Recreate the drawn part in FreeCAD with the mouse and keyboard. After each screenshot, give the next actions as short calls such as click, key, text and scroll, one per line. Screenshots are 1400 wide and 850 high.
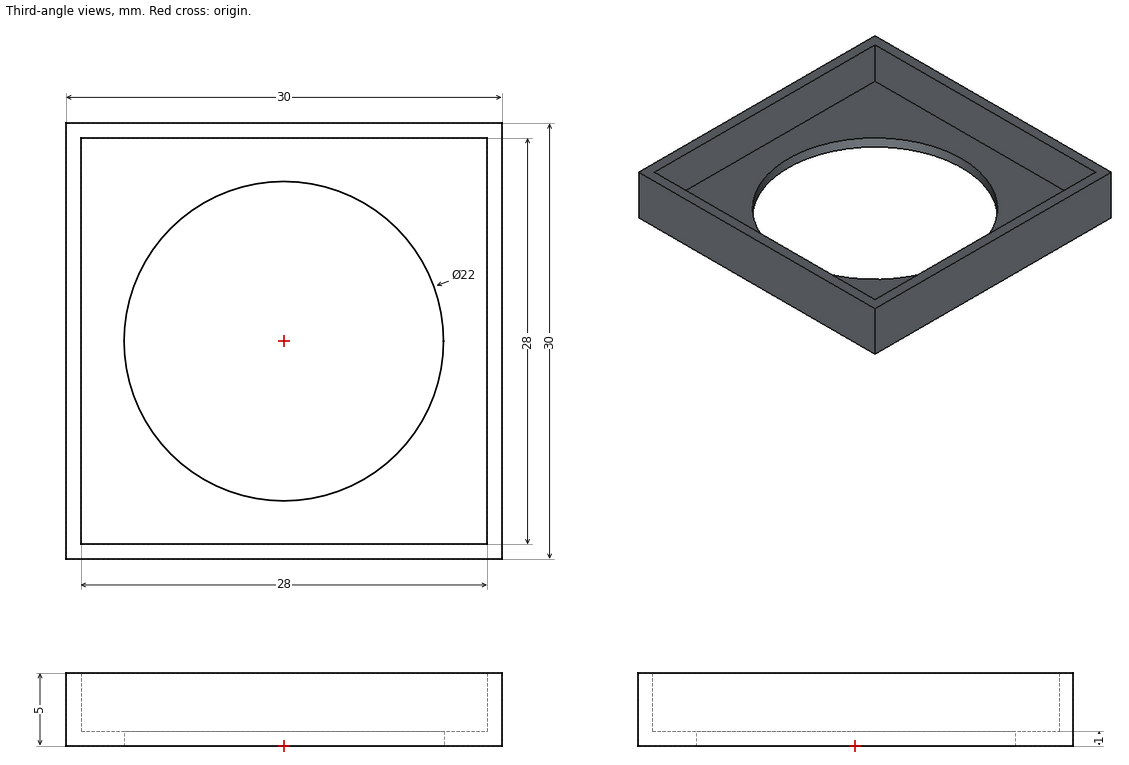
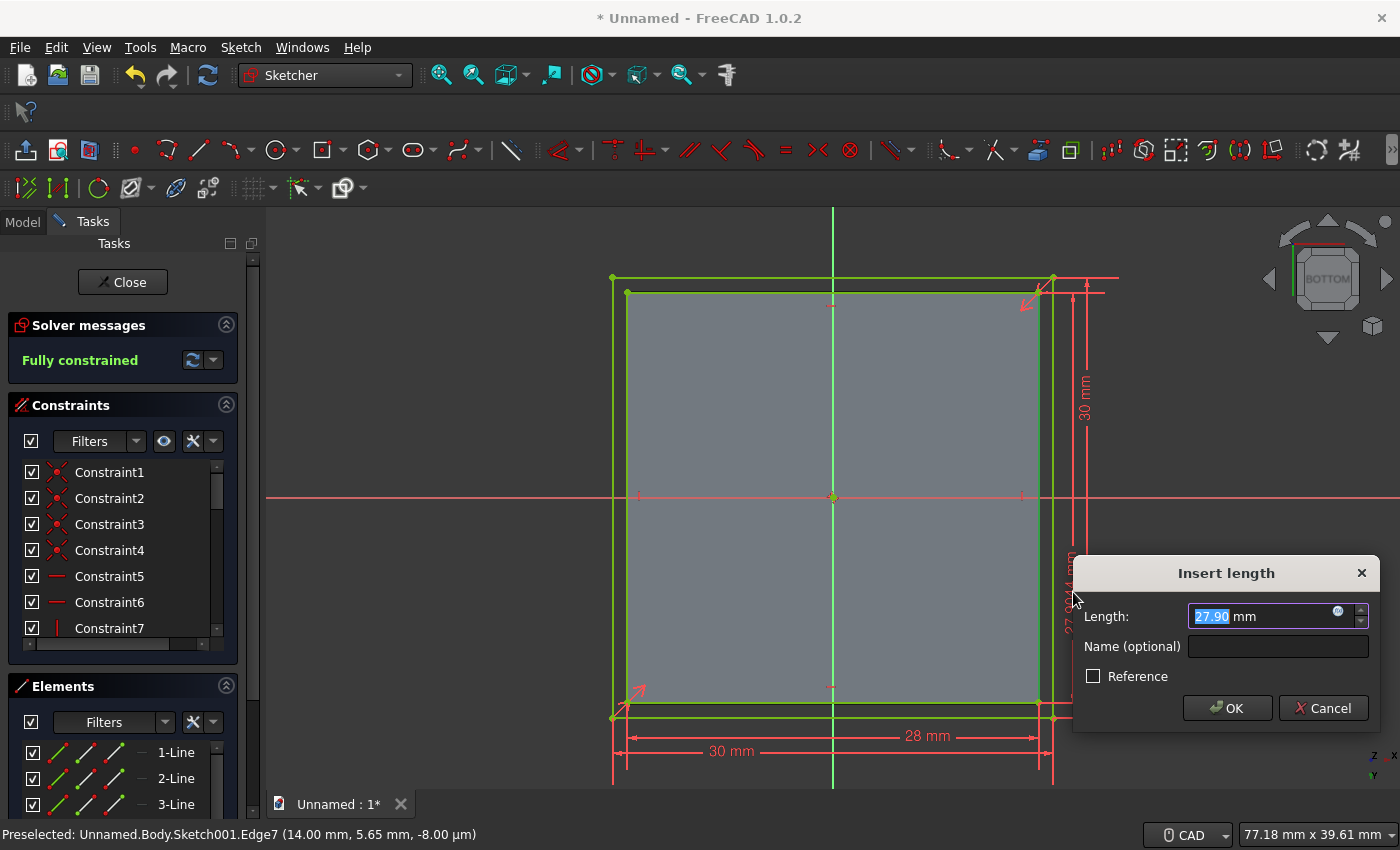
text(28)
key(Return)
key(Escape)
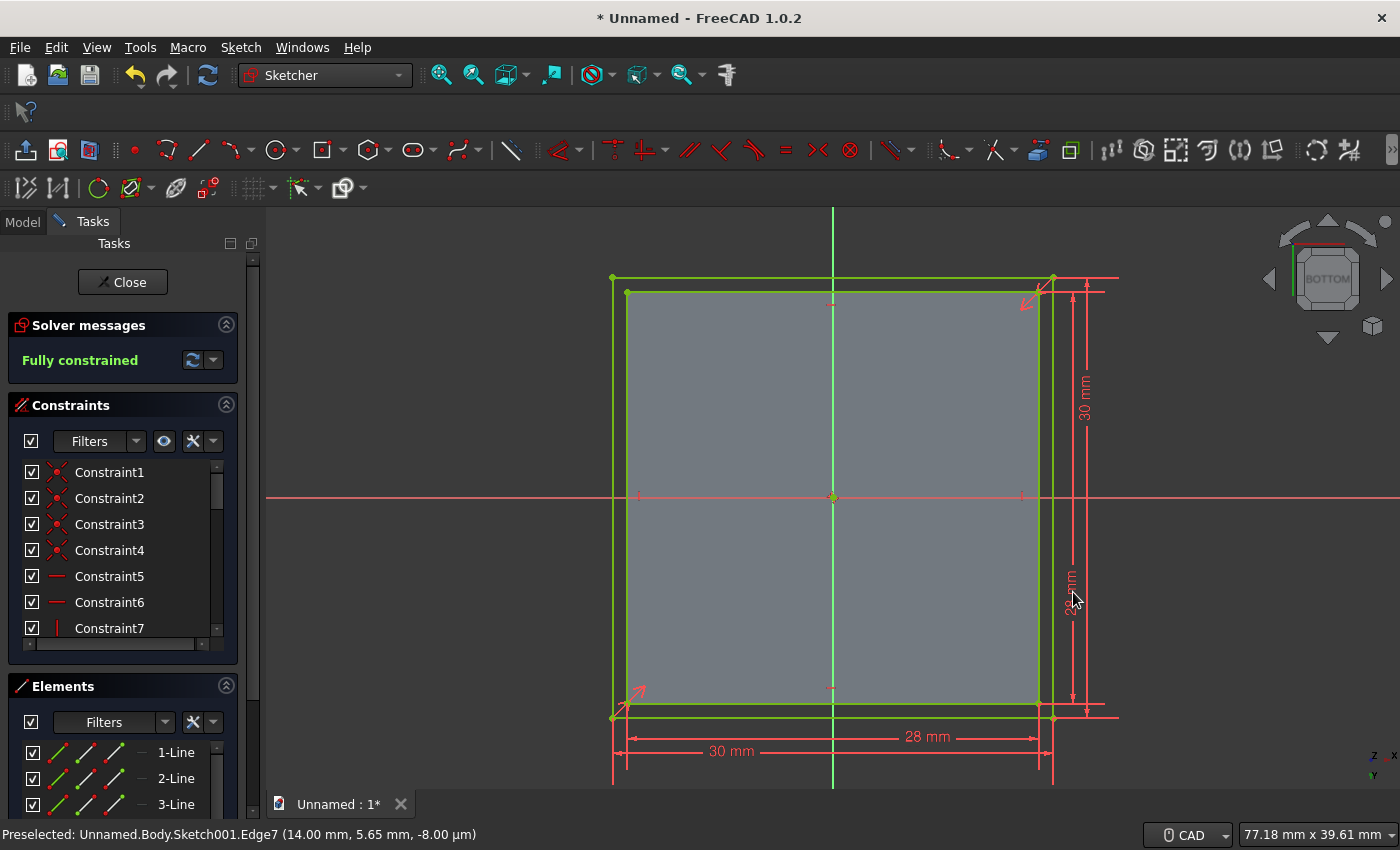
click(123, 282)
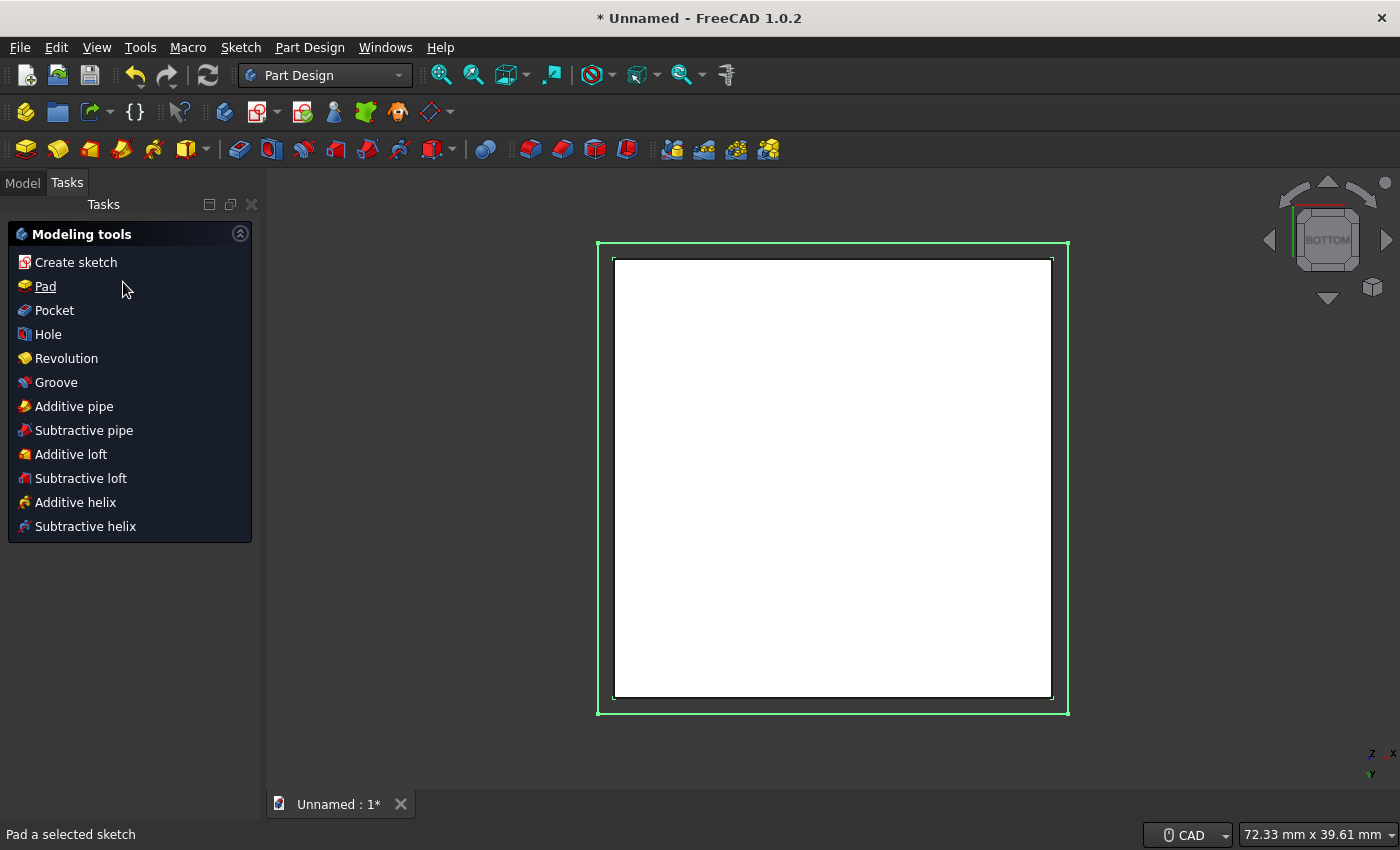
click(26, 150)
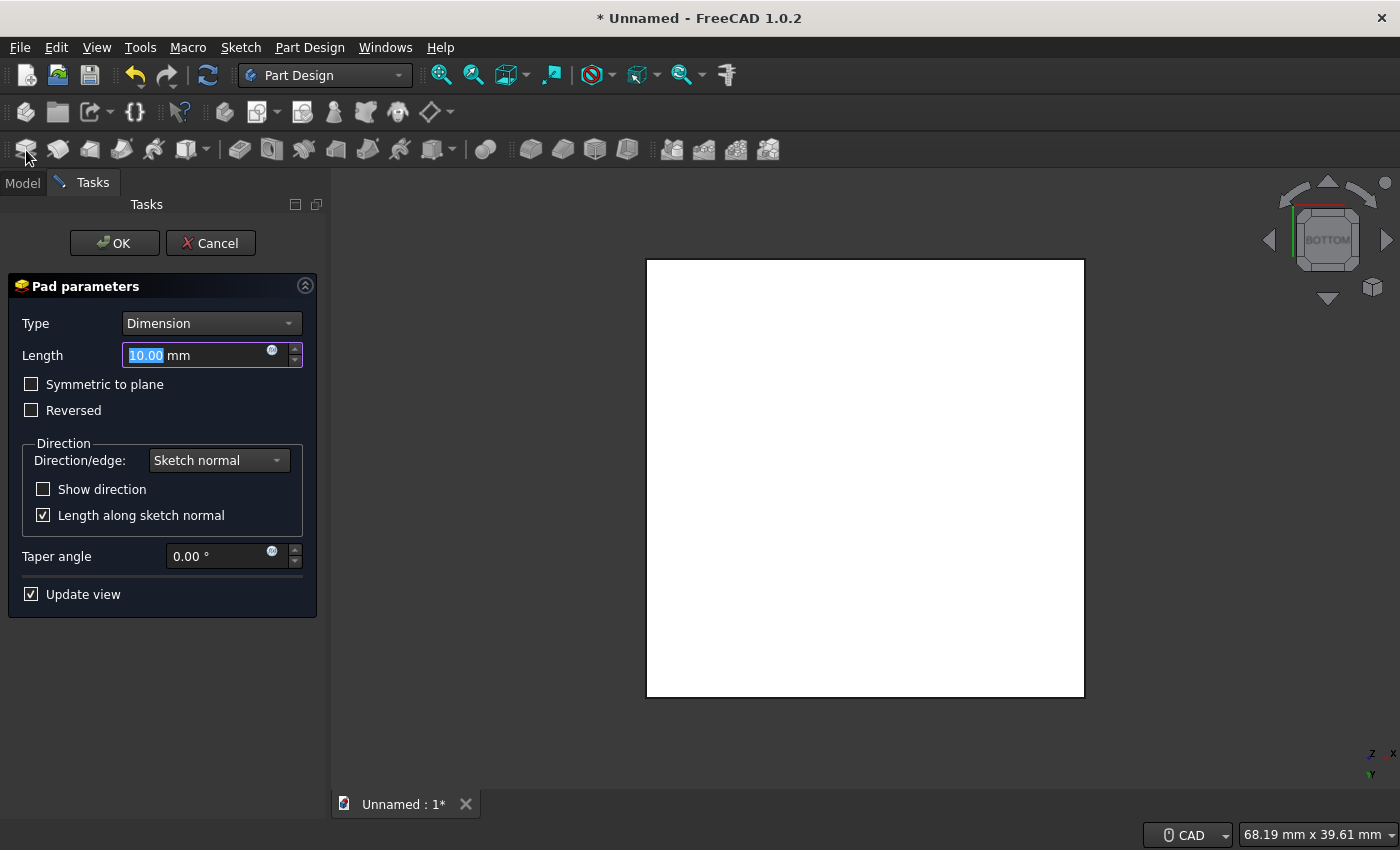
text(5)
key(Tab)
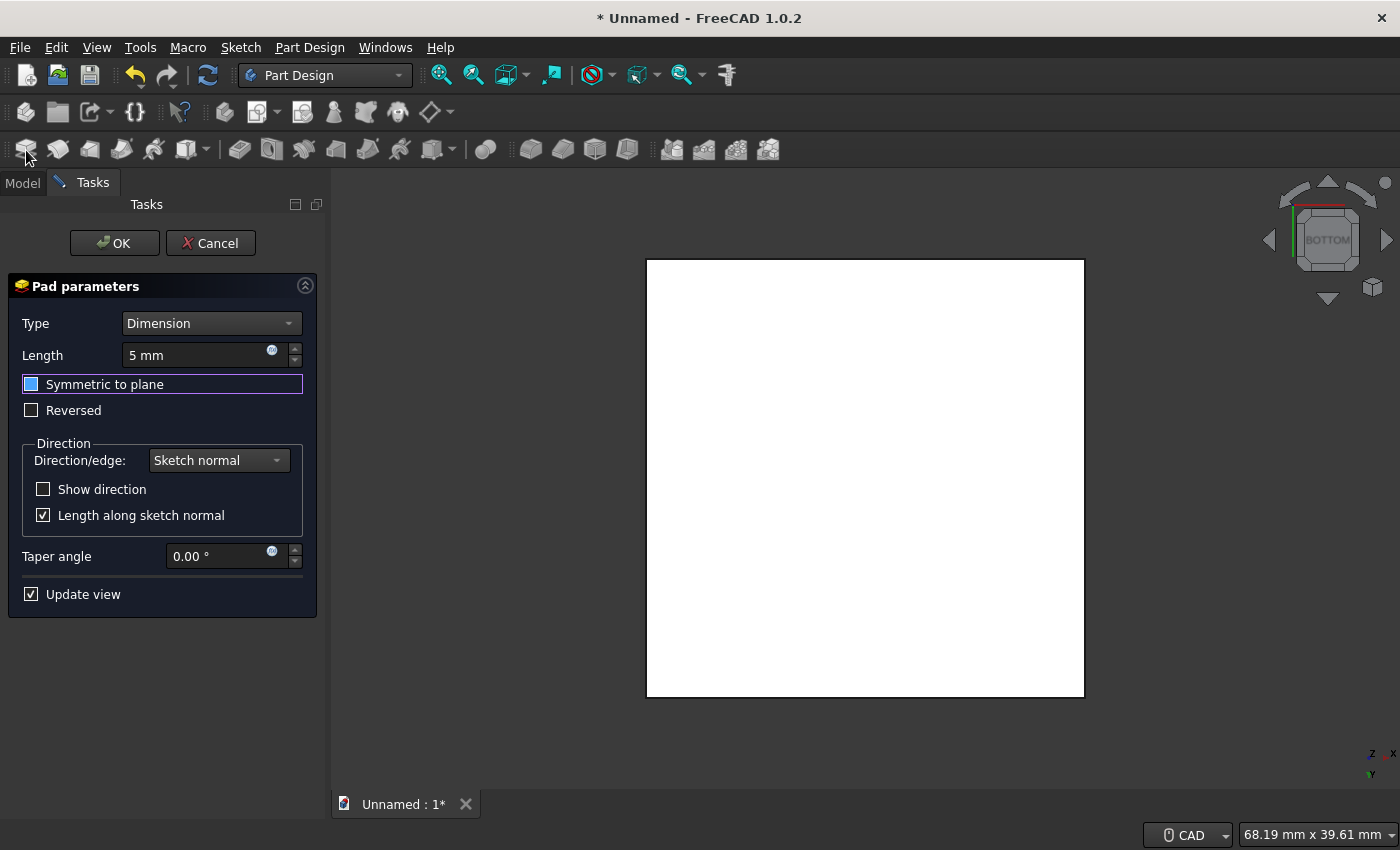
click(30, 410)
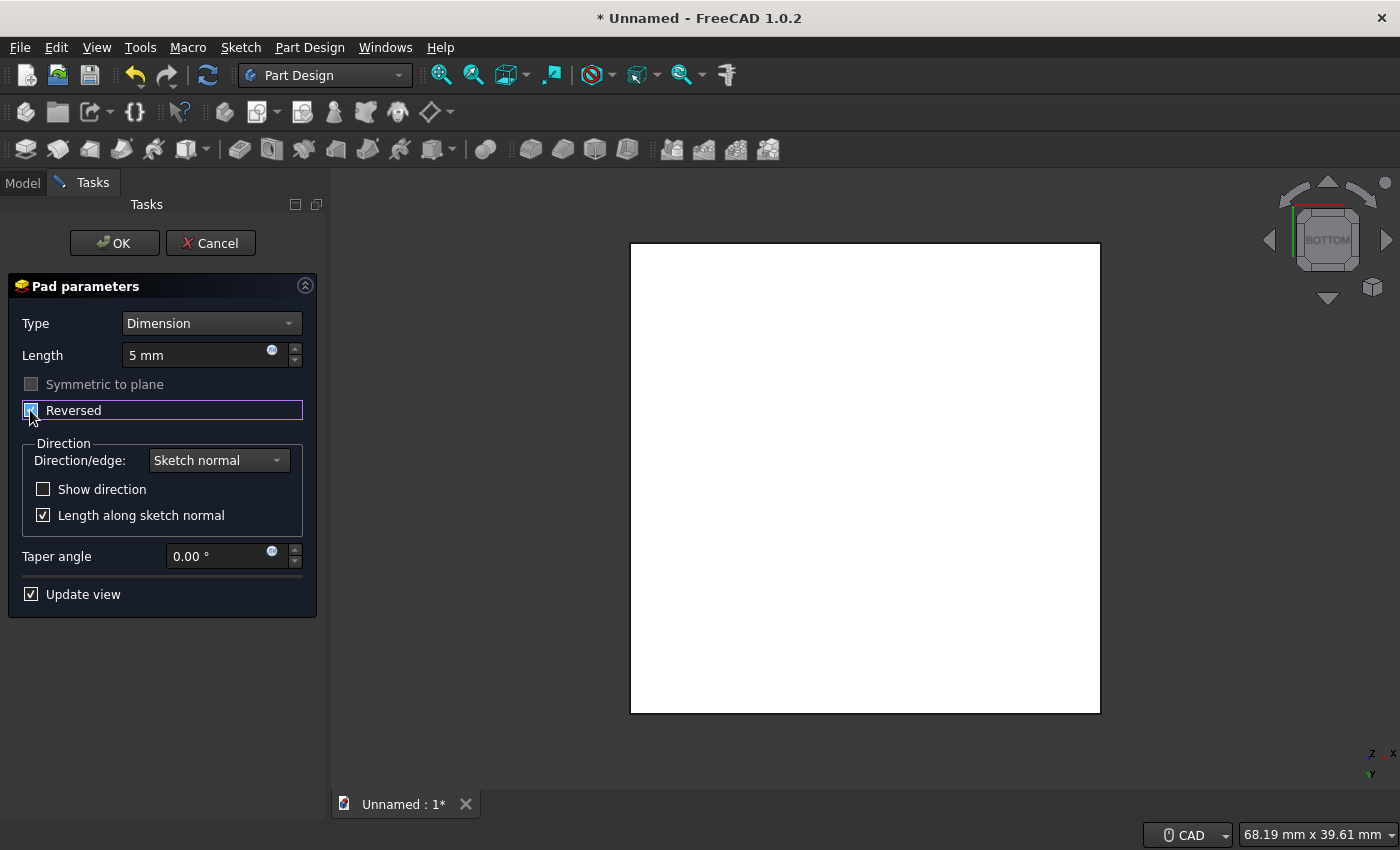
click(115, 243)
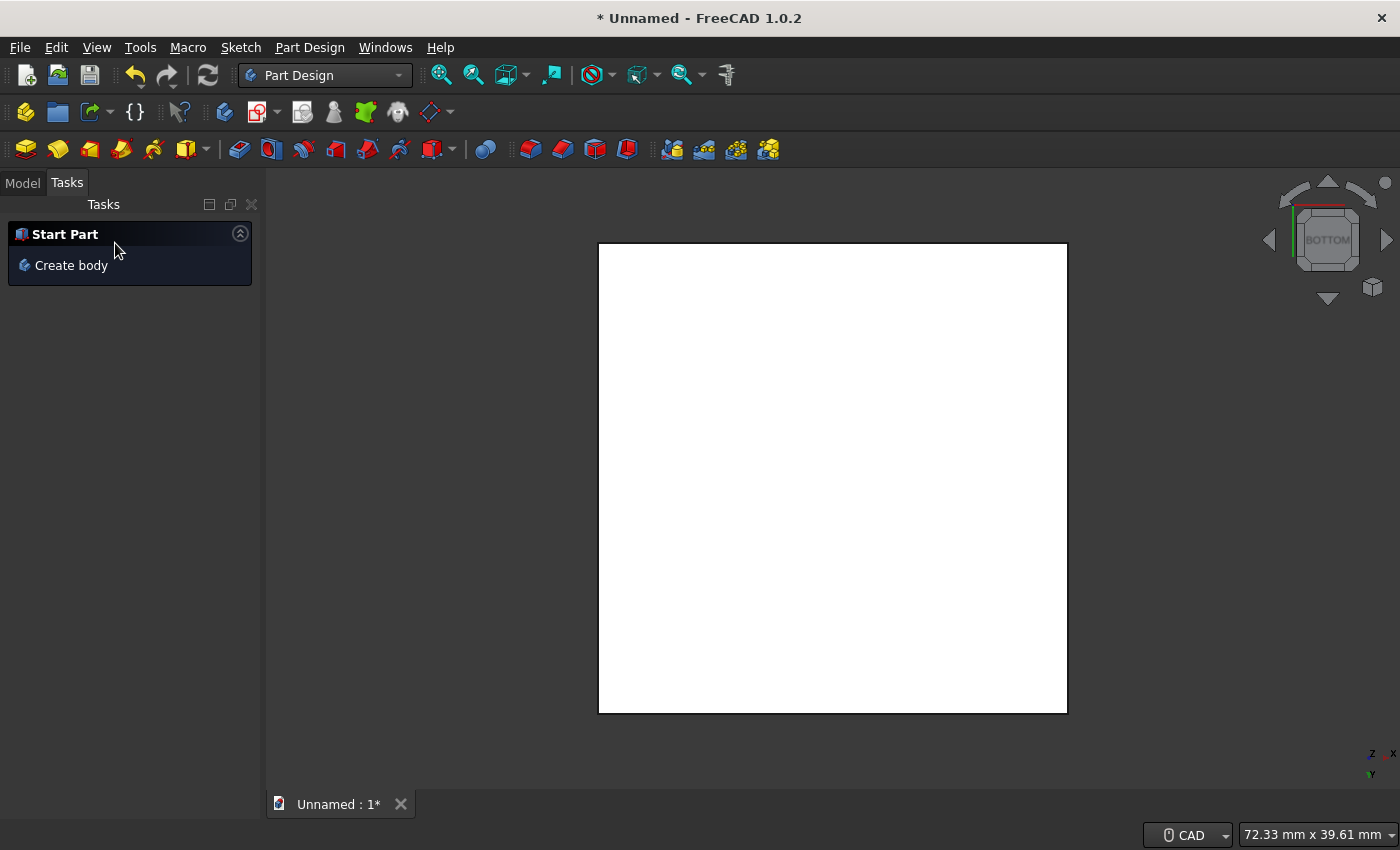
key(0)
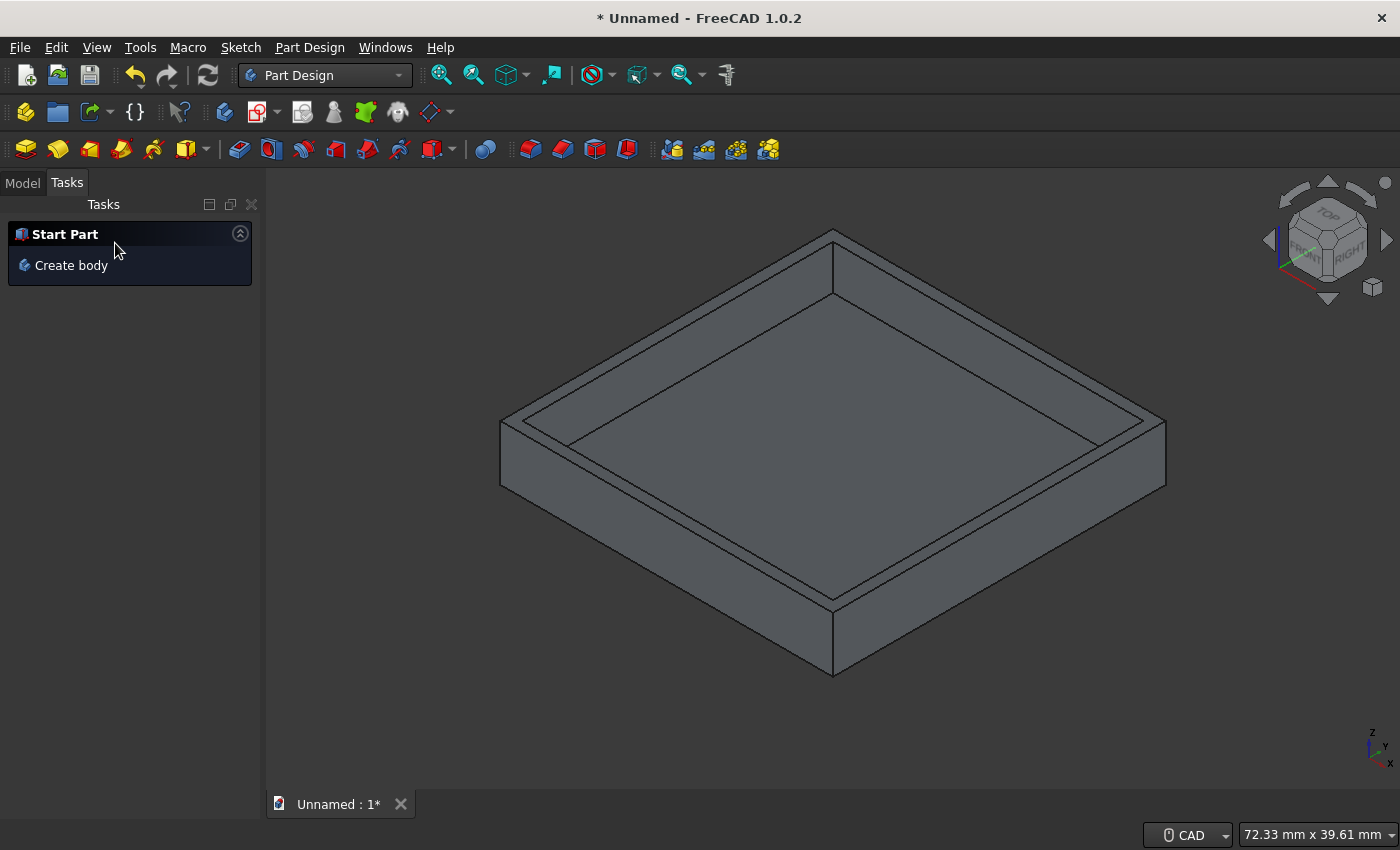
click(833, 471)